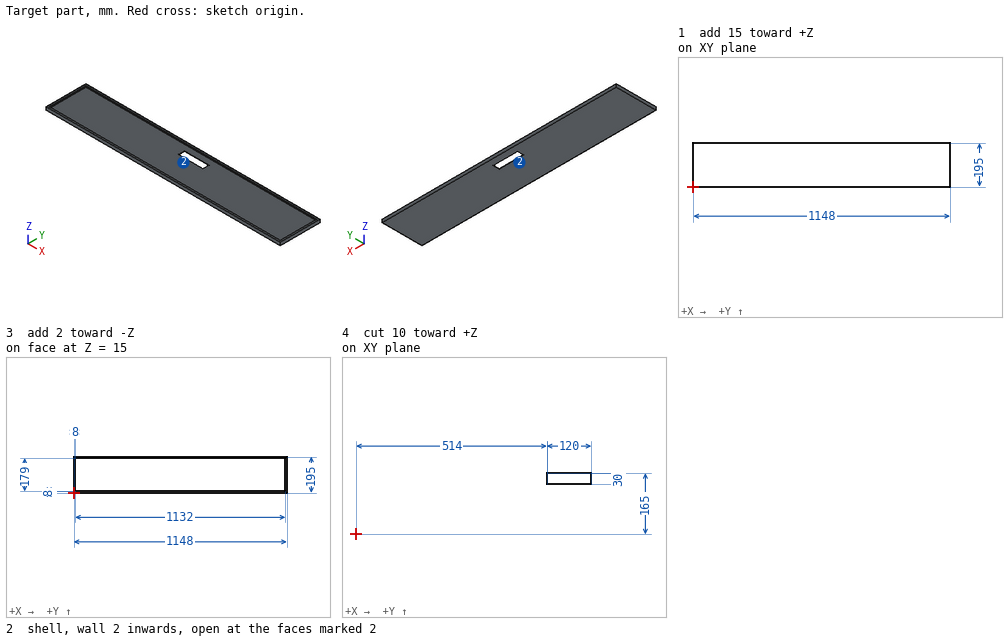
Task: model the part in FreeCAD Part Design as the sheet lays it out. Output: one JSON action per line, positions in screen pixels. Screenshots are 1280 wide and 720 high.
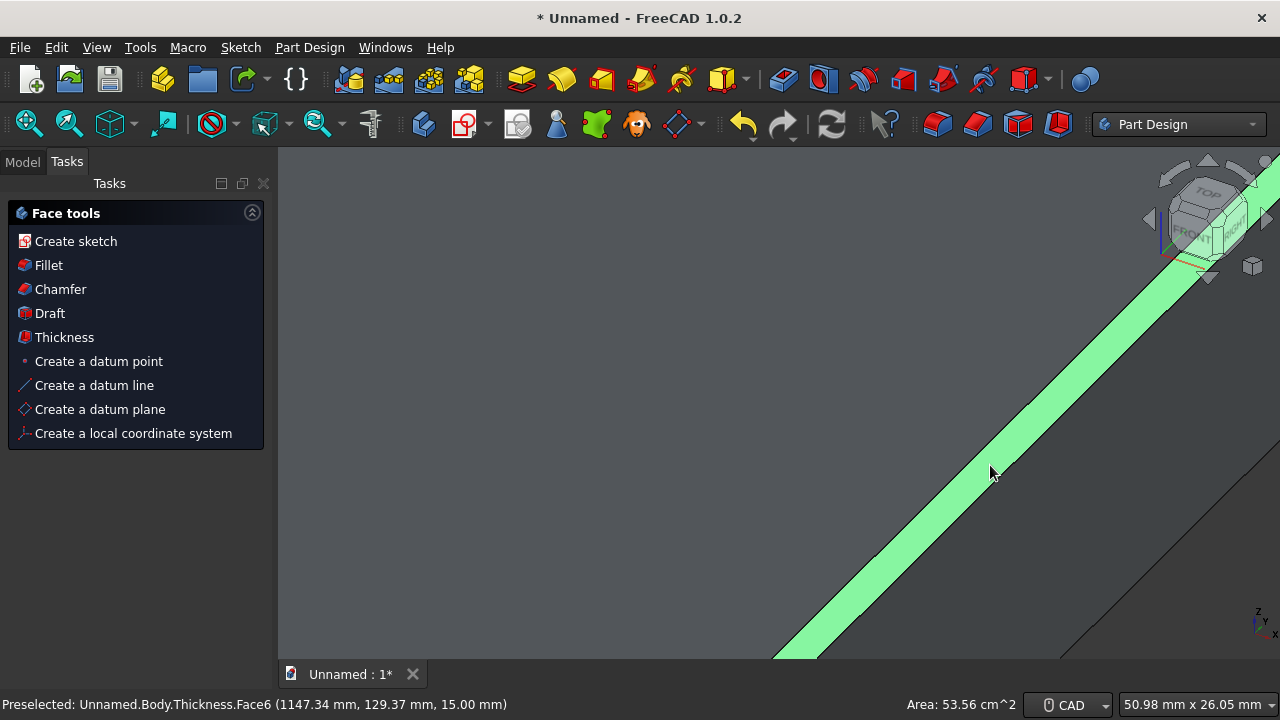
{"action": "left_click", "coordinate": [464, 124]}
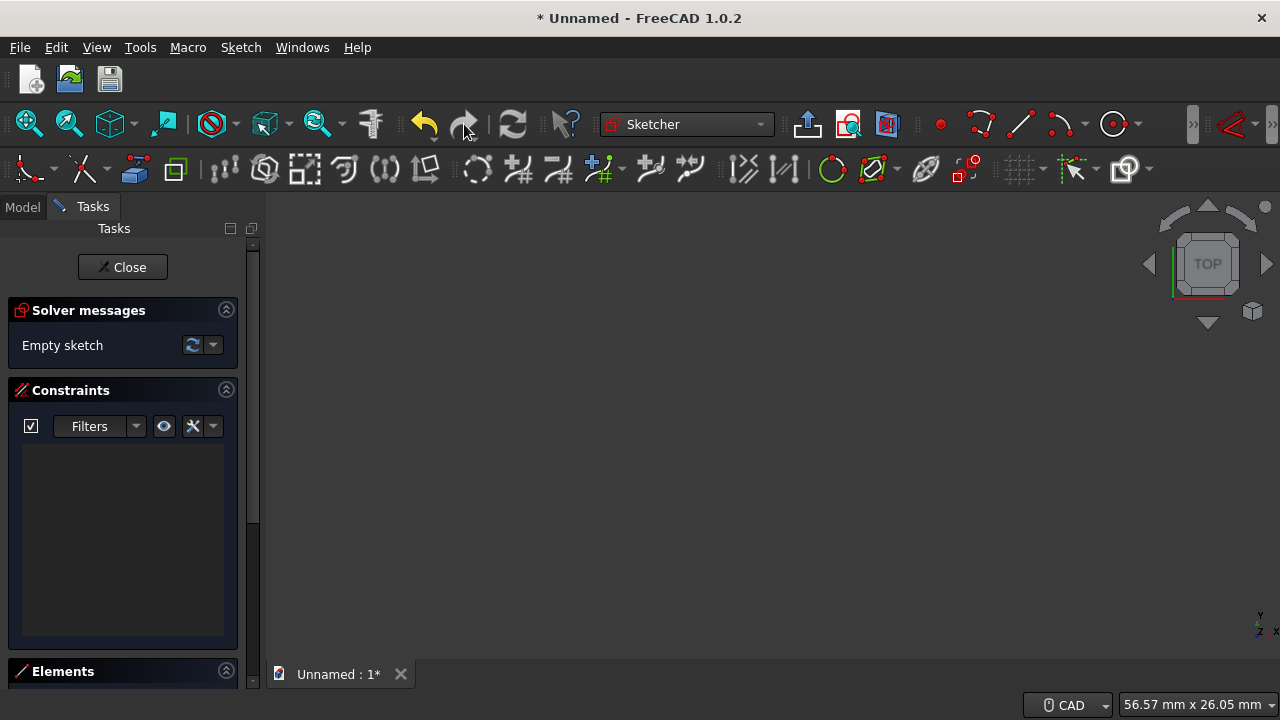
{"action": "scroll", "coordinate": [996, 313], "scroll_direction": "down", "scroll_amount": 17}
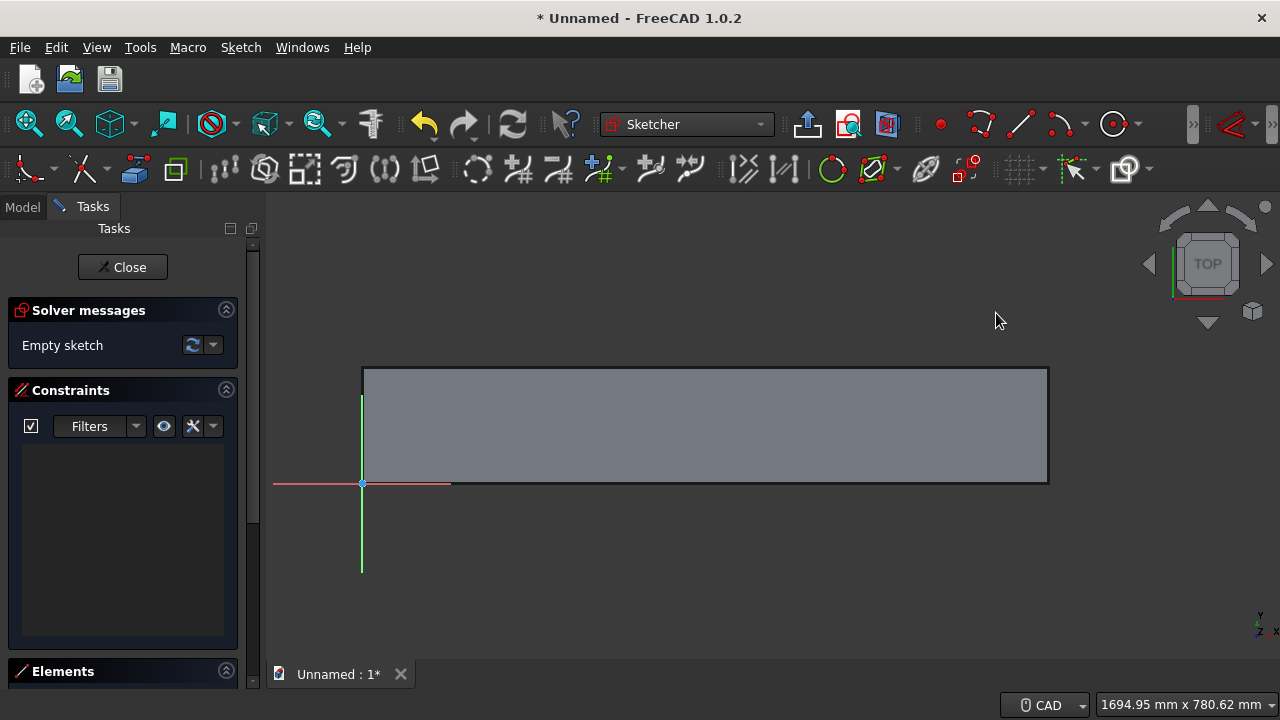
{"action": "key", "text": "g r"}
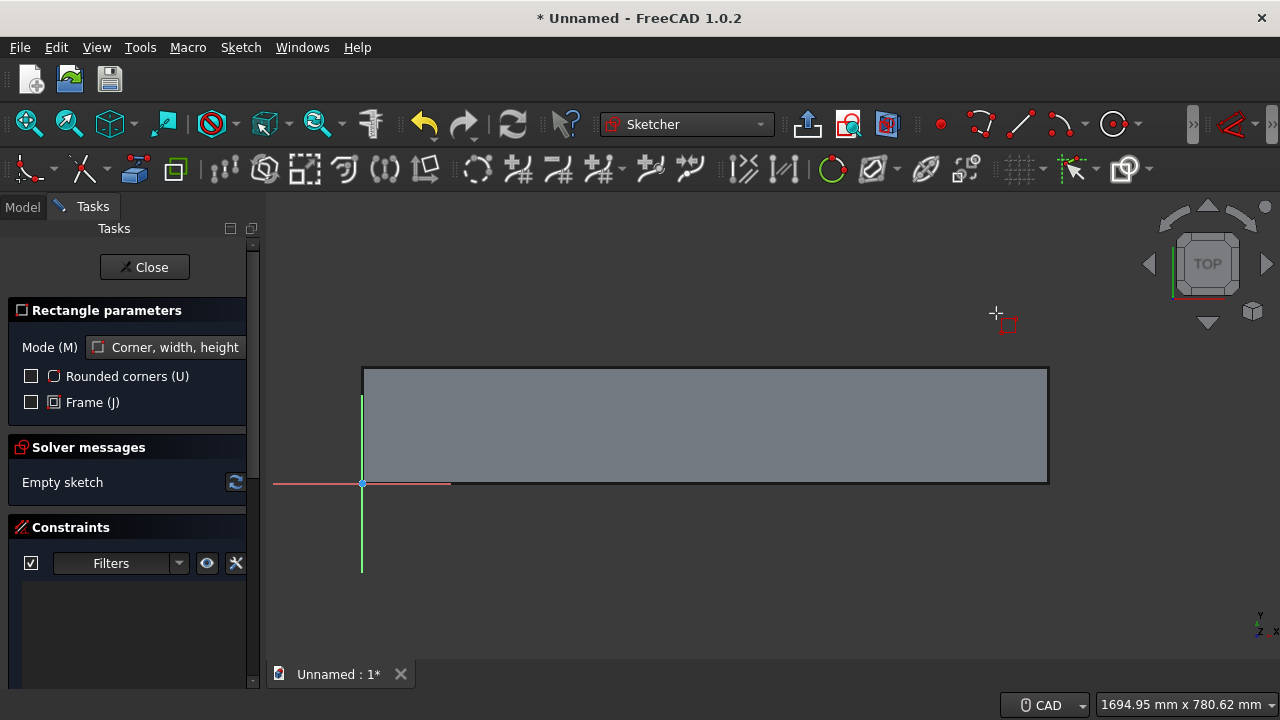
{"action": "left_click", "coordinate": [362, 484]}
{"action": "mouse_move", "coordinate": [1049, 367]}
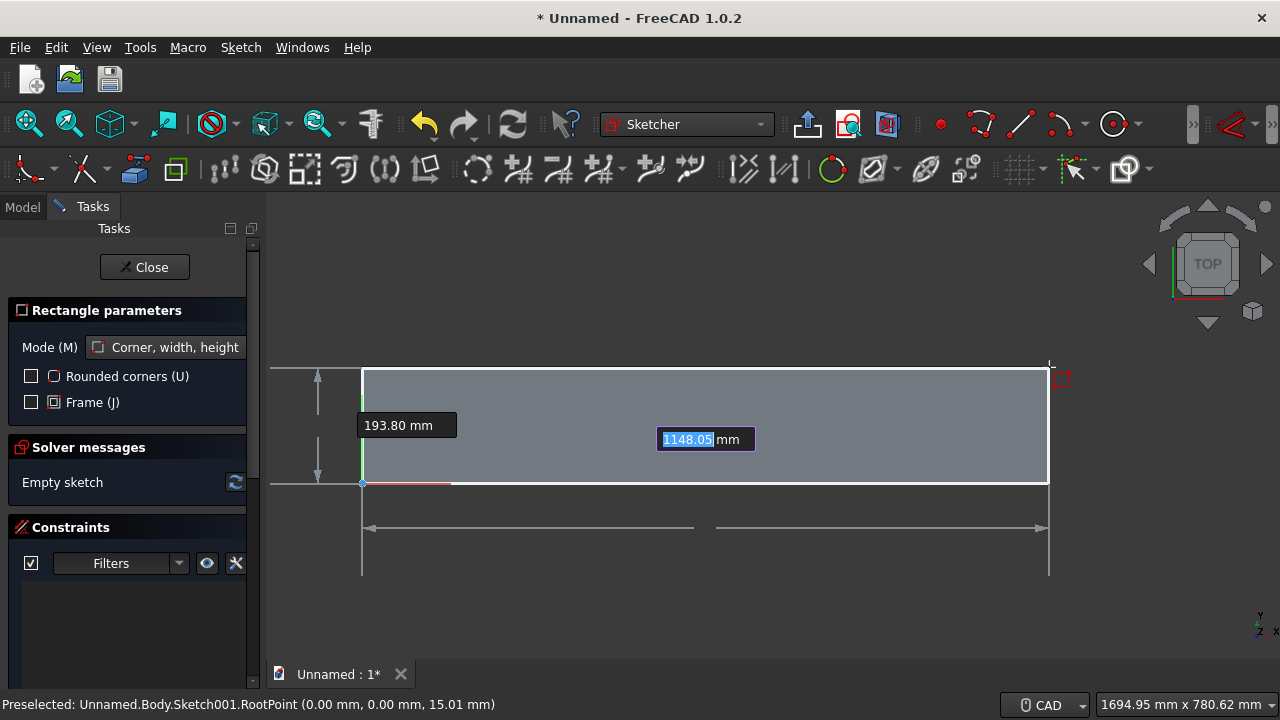
{"action": "type", "text": "1148"}
{"action": "key", "text": "Tab"}
{"action": "type", "text": "195"}
{"action": "key", "text": "Return"}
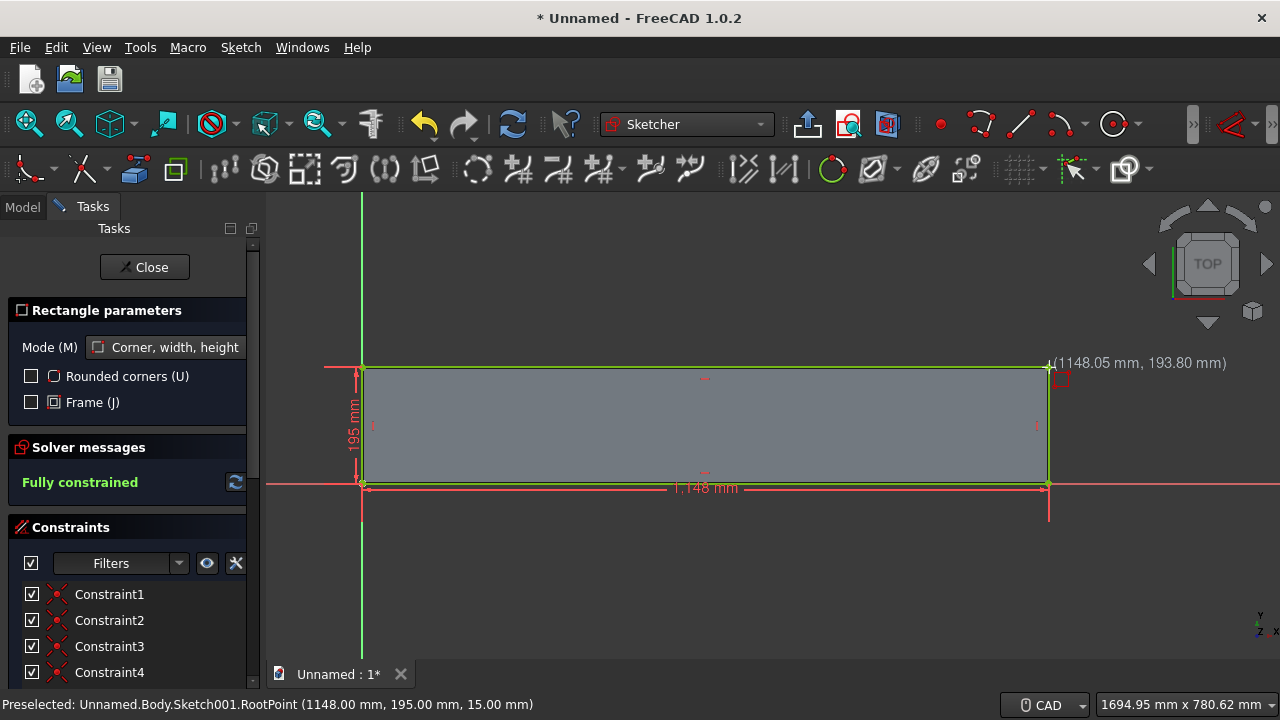
{"action": "scroll", "coordinate": [367, 372], "scroll_direction": "up", "scroll_amount": 6}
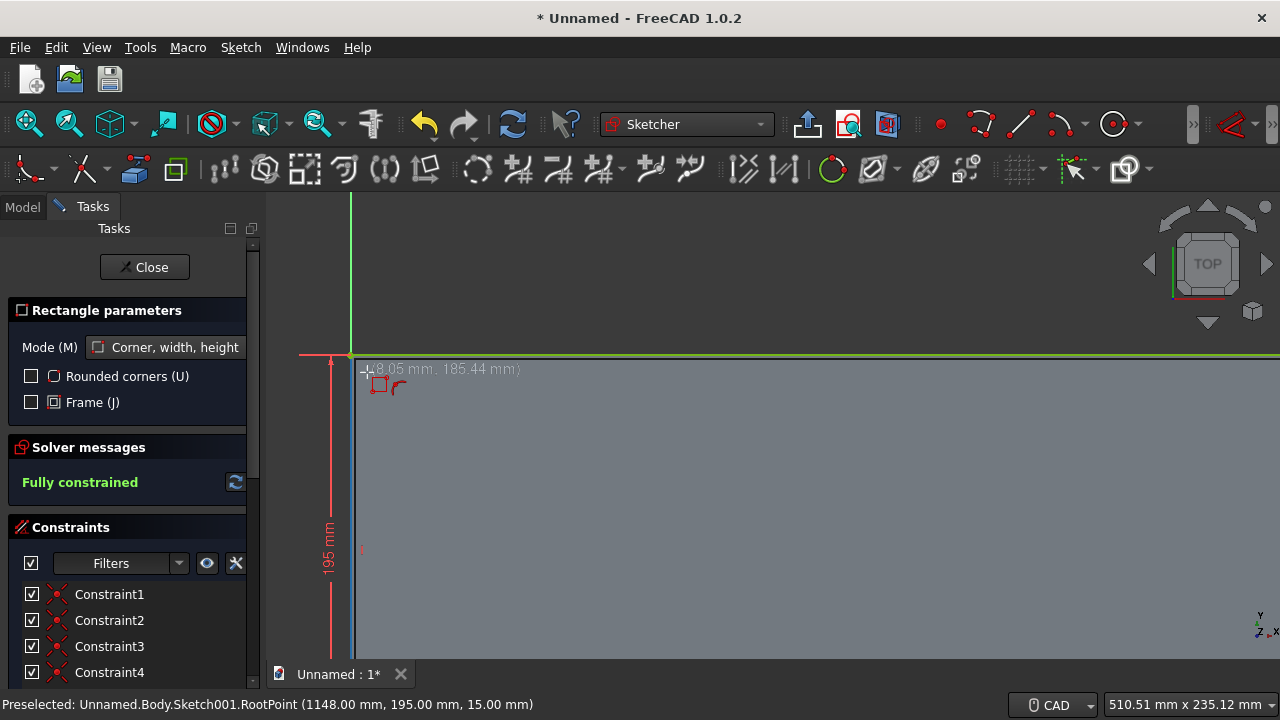
{"action": "left_click", "coordinate": [367, 371]}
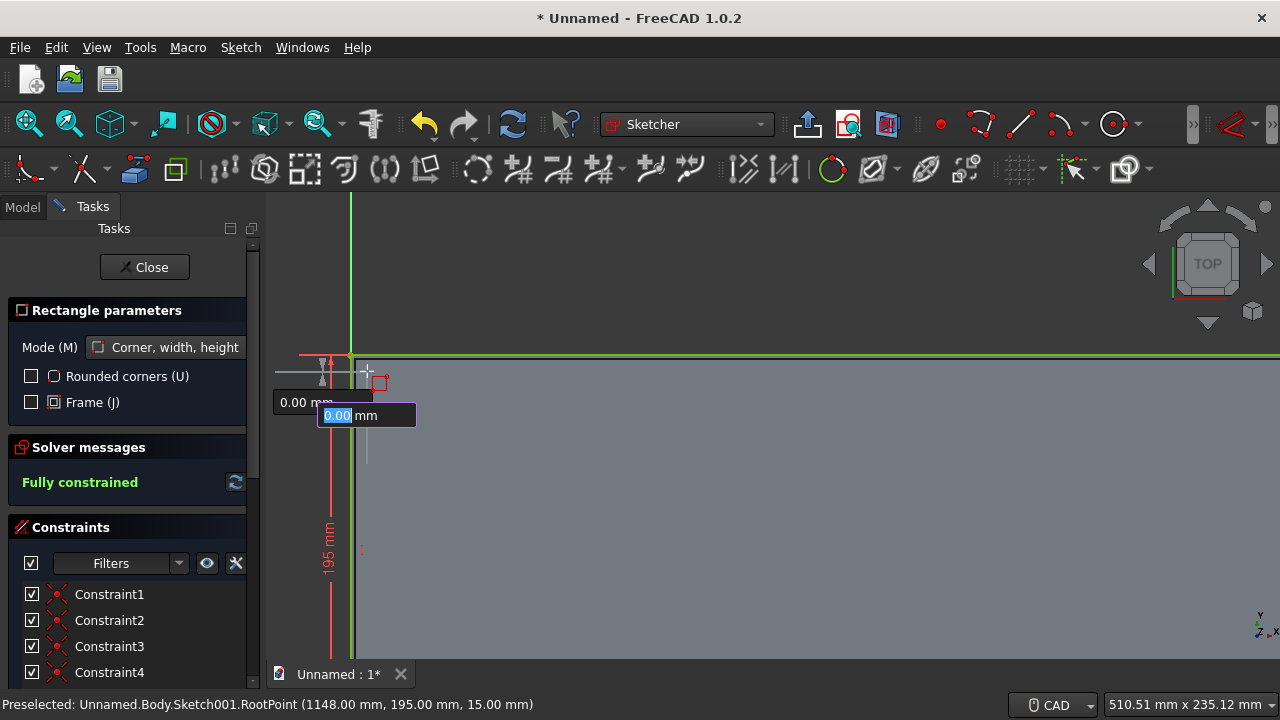
{"action": "scroll", "coordinate": [447, 385], "scroll_direction": "down", "scroll_amount": 7}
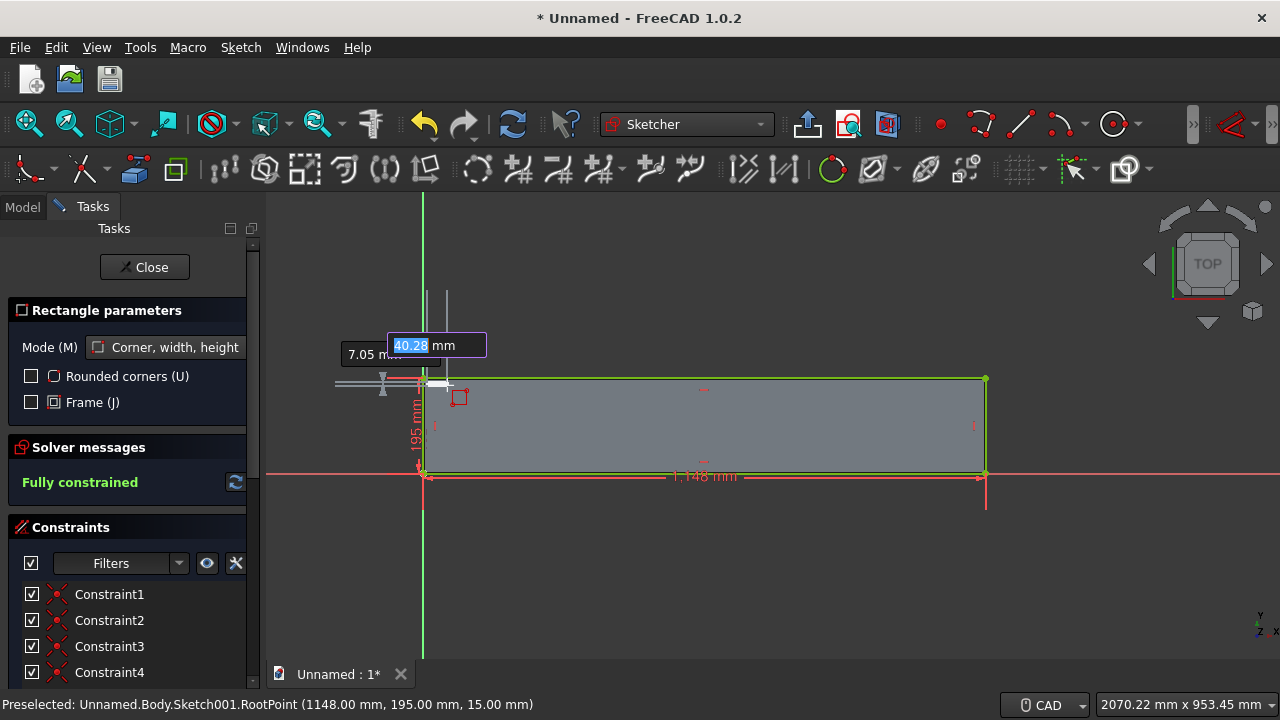
{"action": "scroll", "coordinate": [982, 470], "scroll_direction": "up", "scroll_amount": 7}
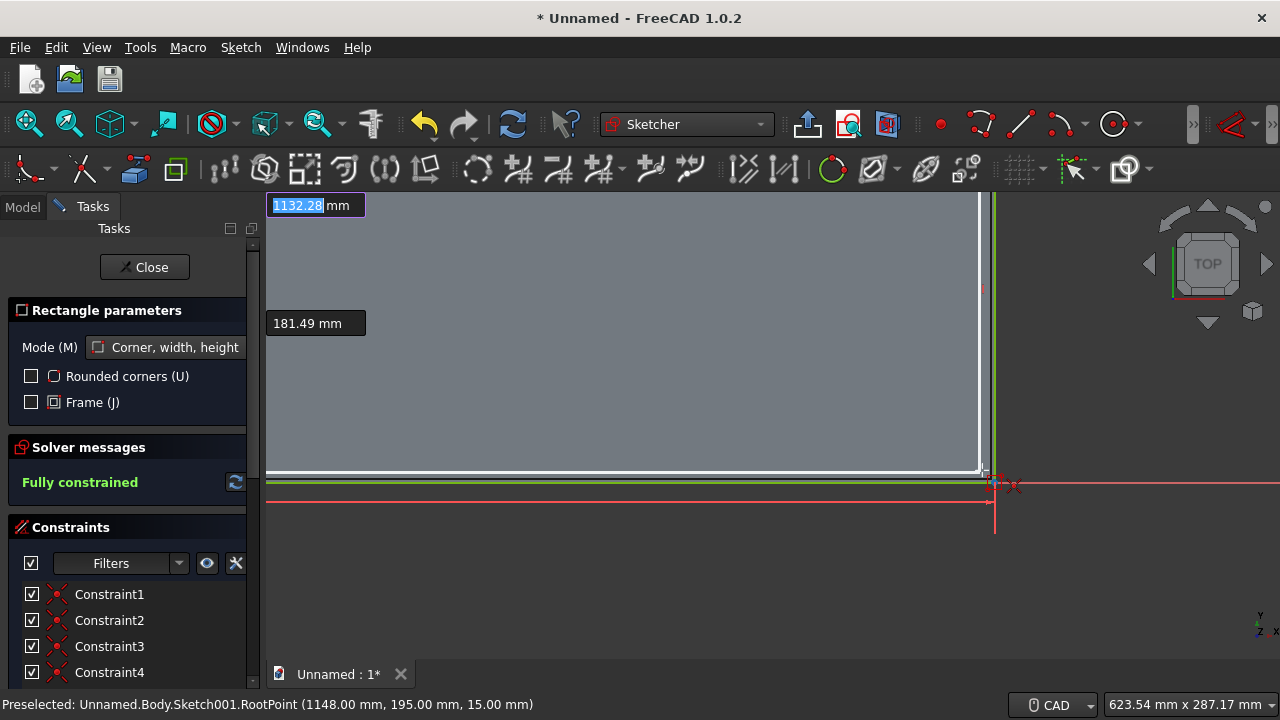
{"action": "left_click", "coordinate": [979, 467]}
{"action": "key", "text": "Escape"}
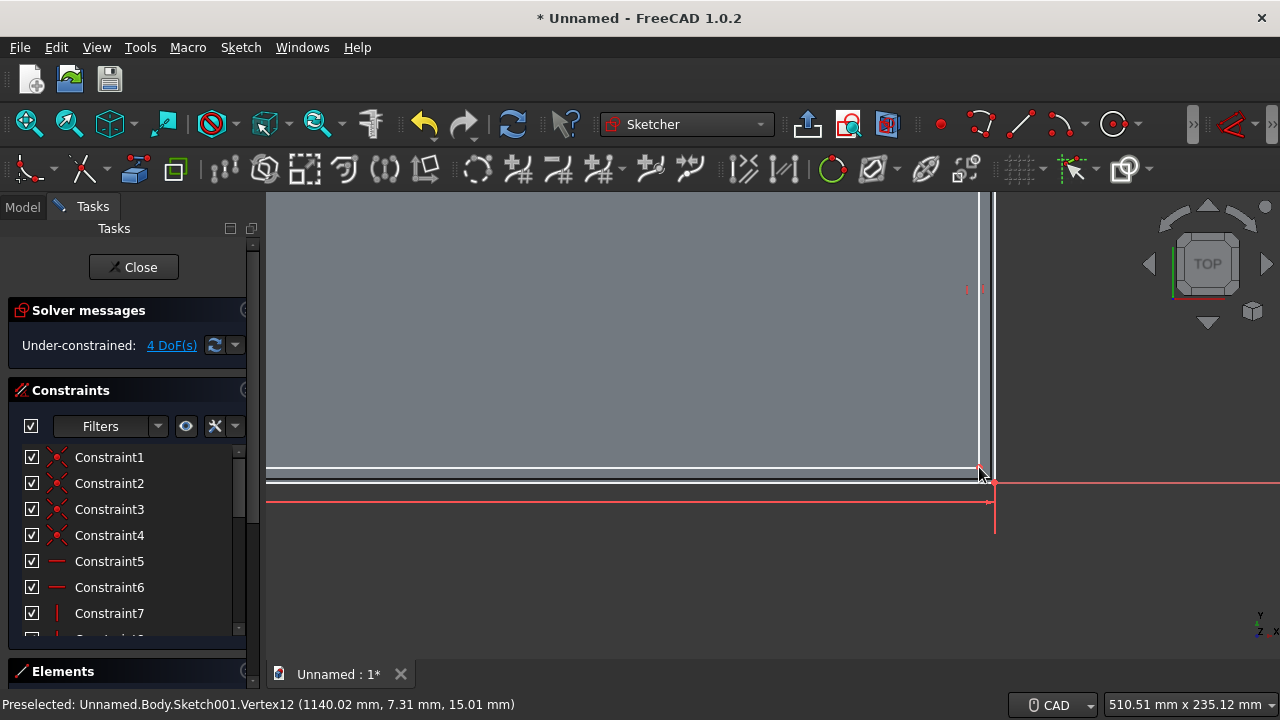
{"action": "left_click", "coordinate": [1232, 124]}